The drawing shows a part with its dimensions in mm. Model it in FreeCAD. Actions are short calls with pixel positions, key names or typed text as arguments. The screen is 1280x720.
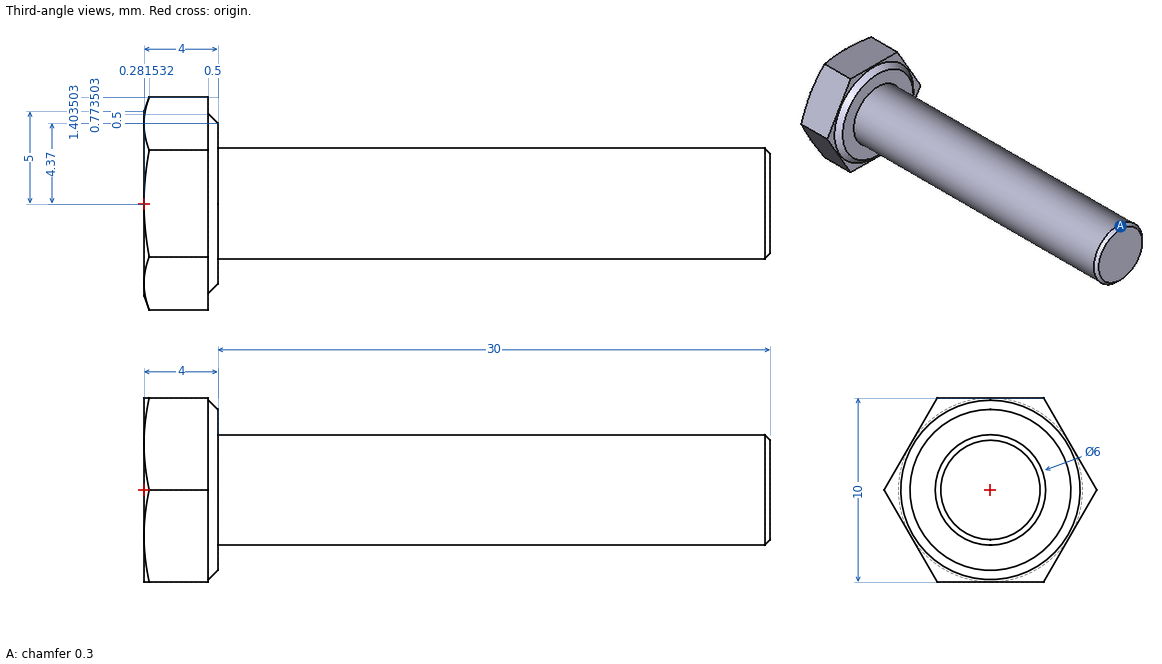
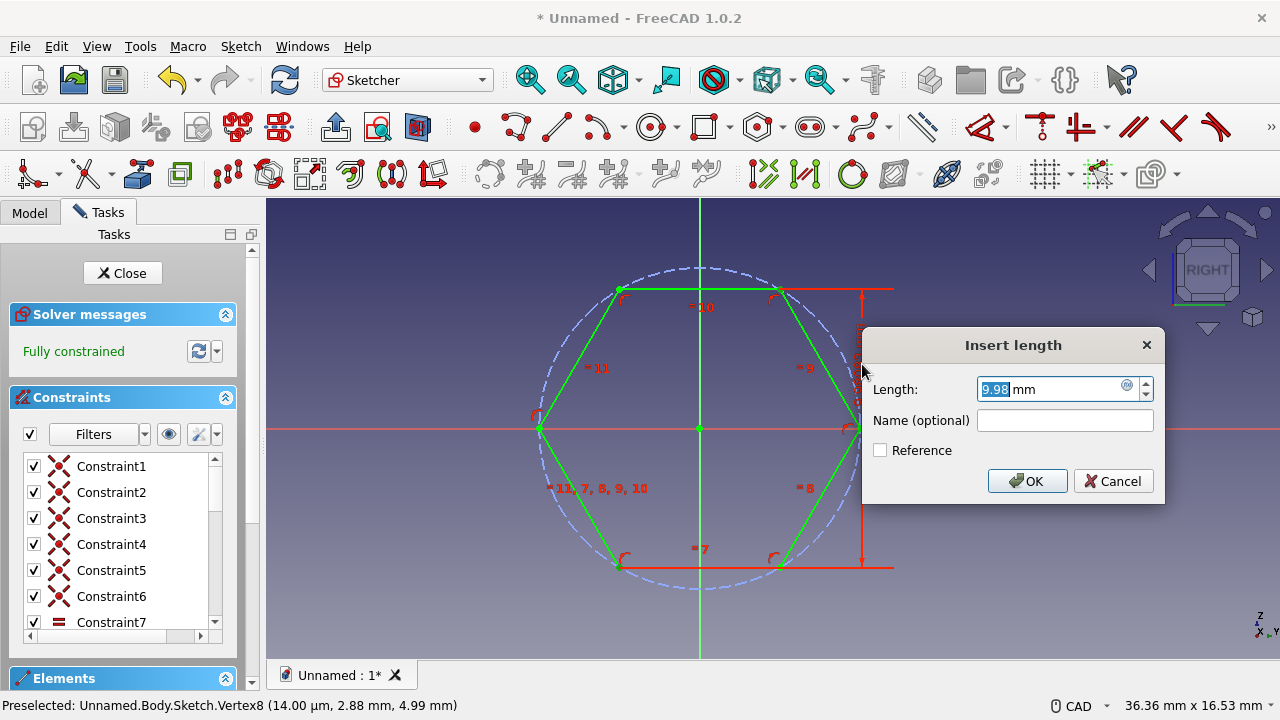
text(10)
key(Return)
key(Escape)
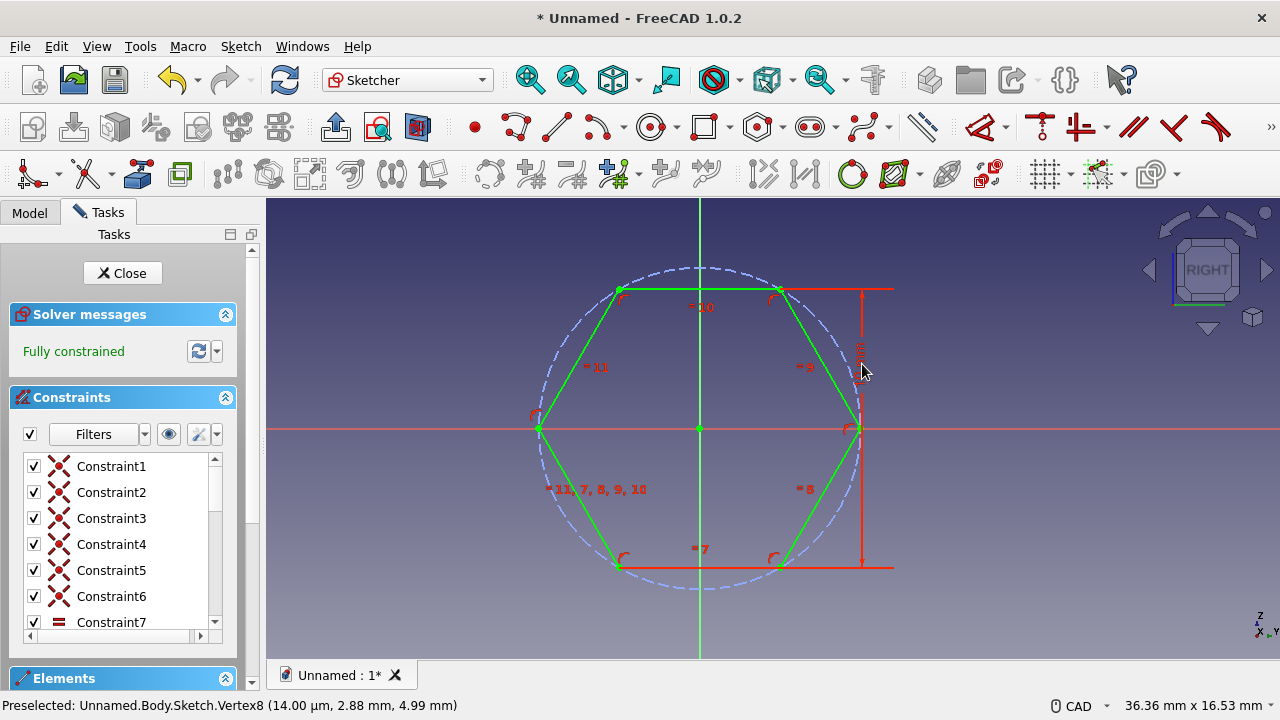
click(123, 273)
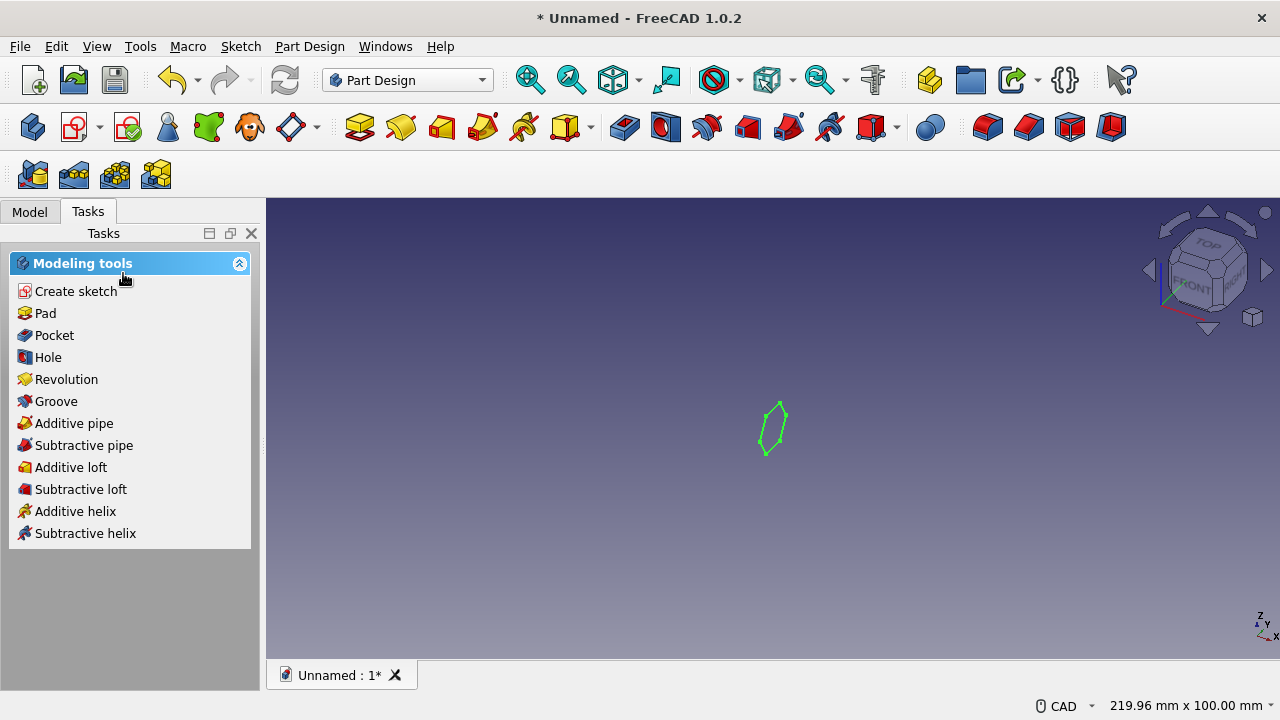
click(360, 128)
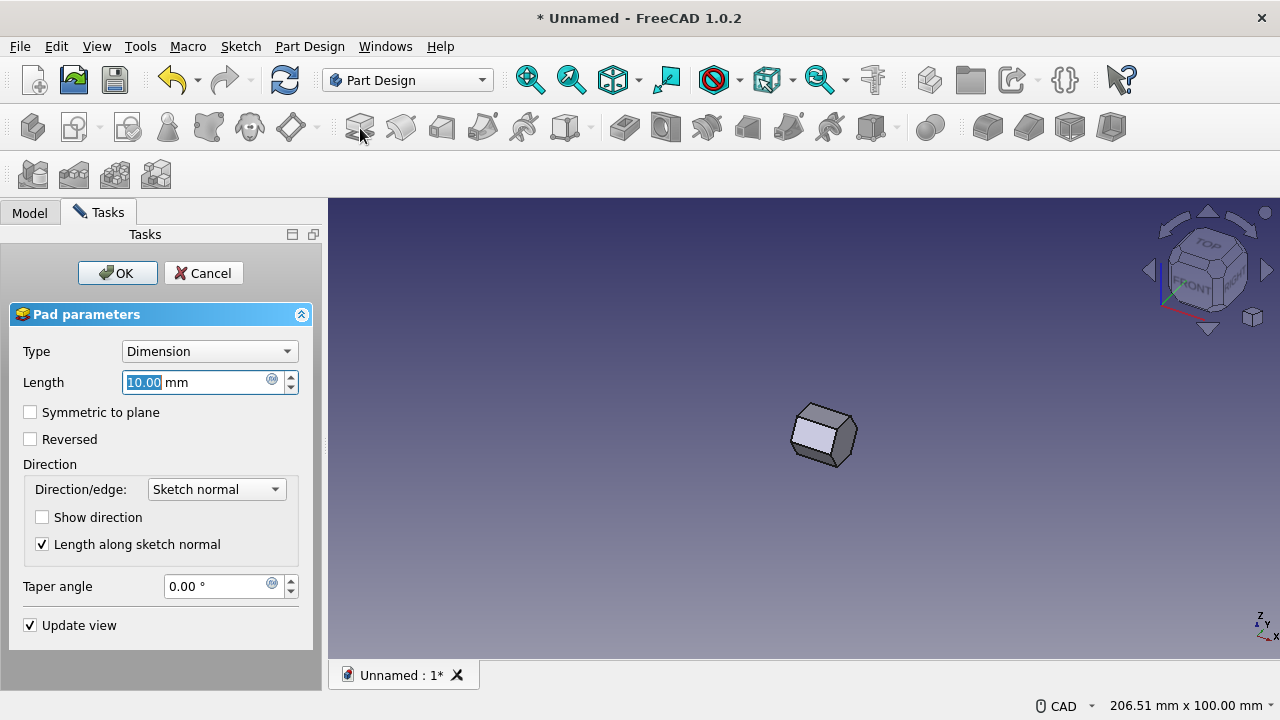
text(4)
key(Tab)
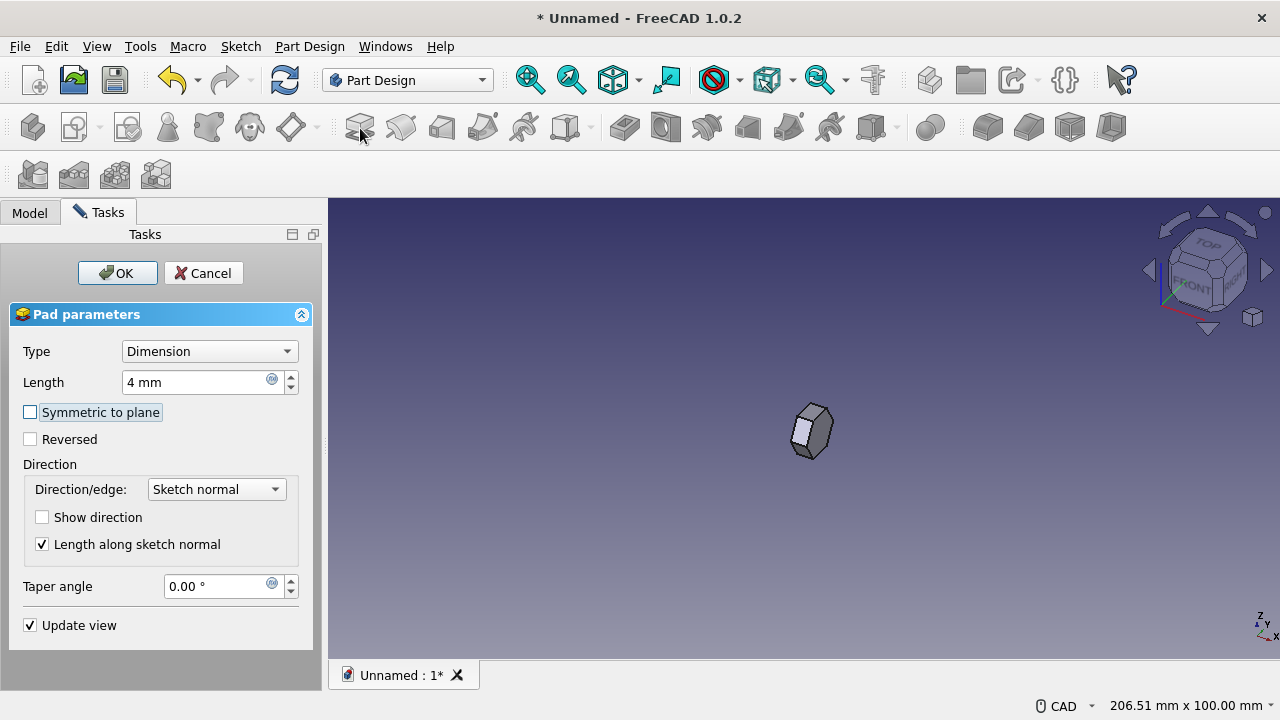
click(118, 273)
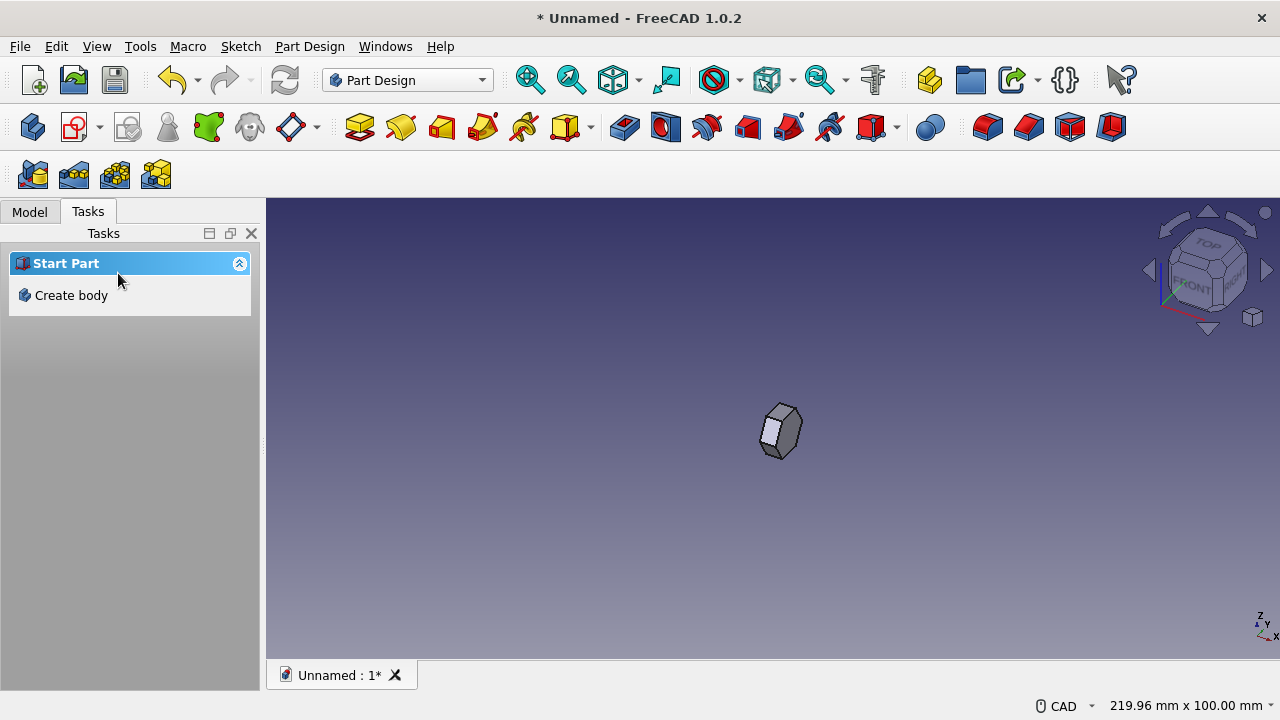
click(531, 80)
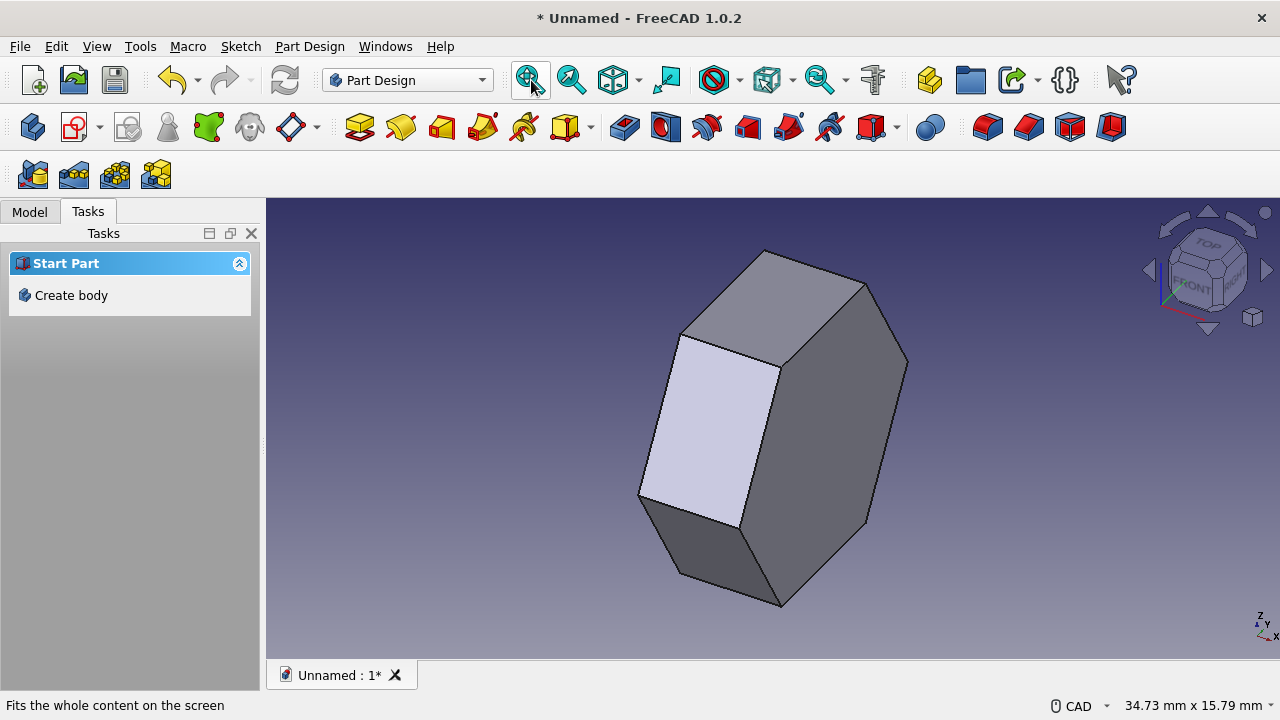
click(74, 128)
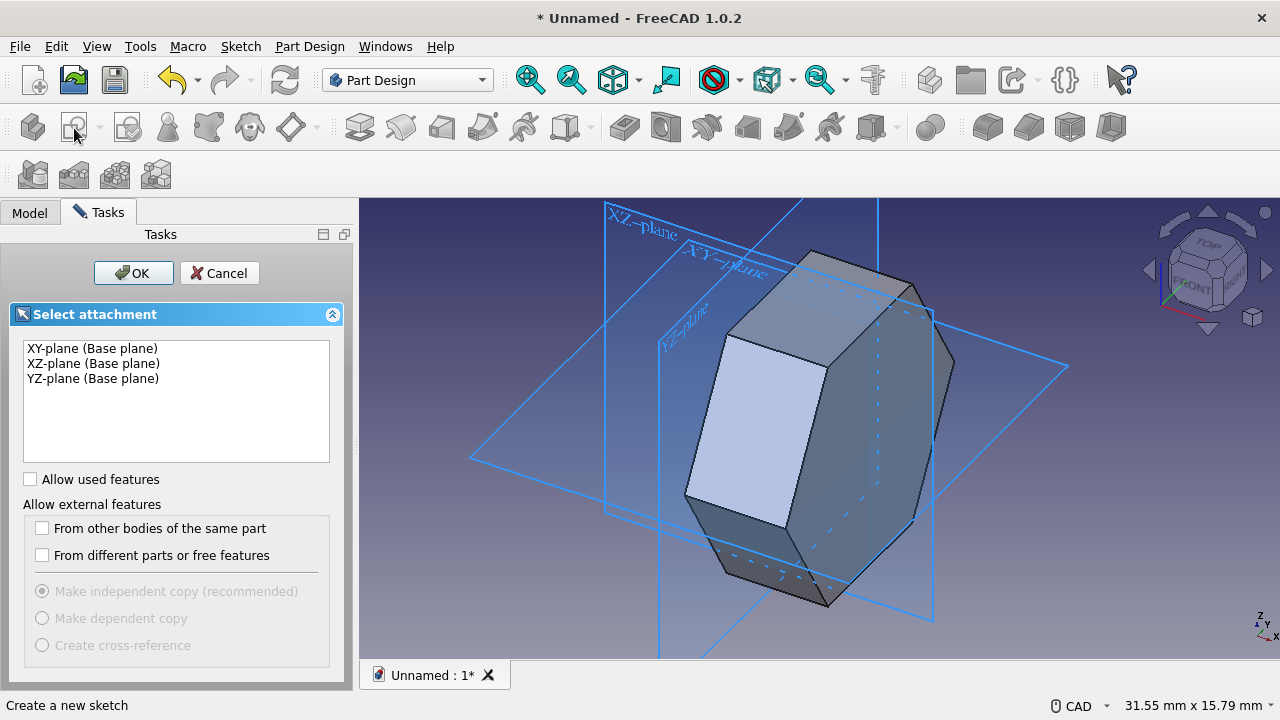
click(84, 348)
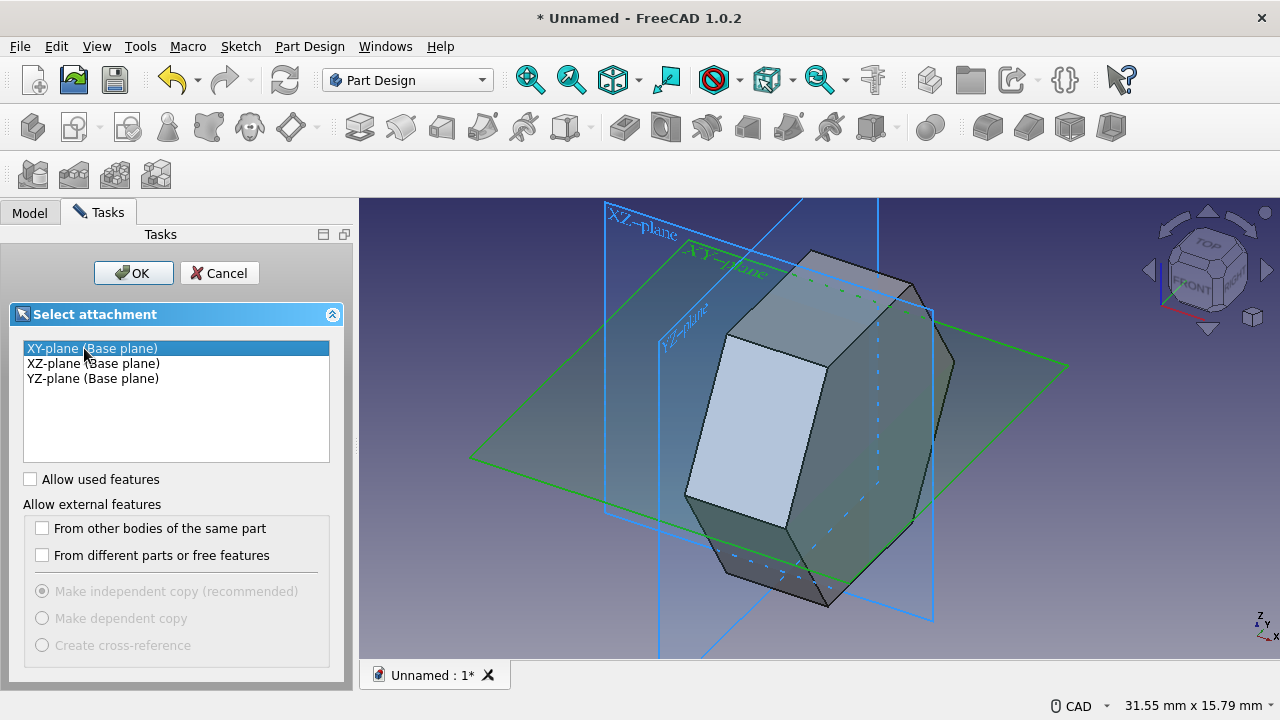
click(134, 273)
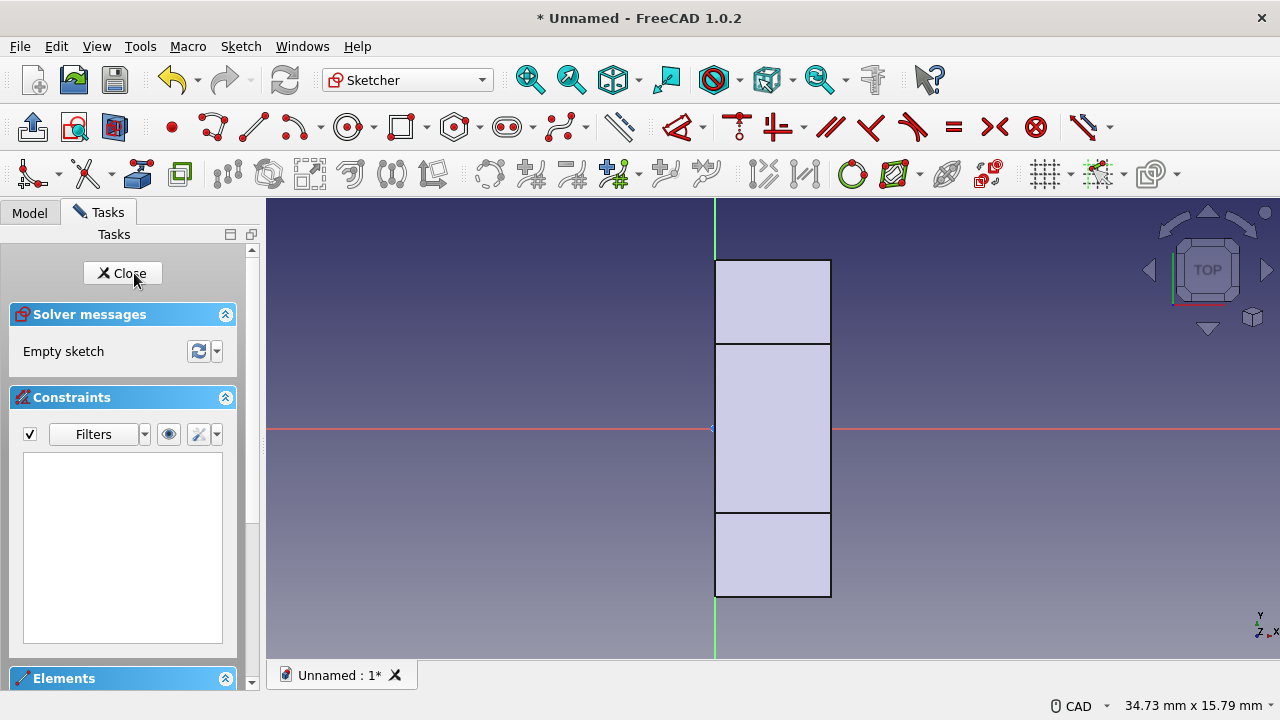
click(115, 128)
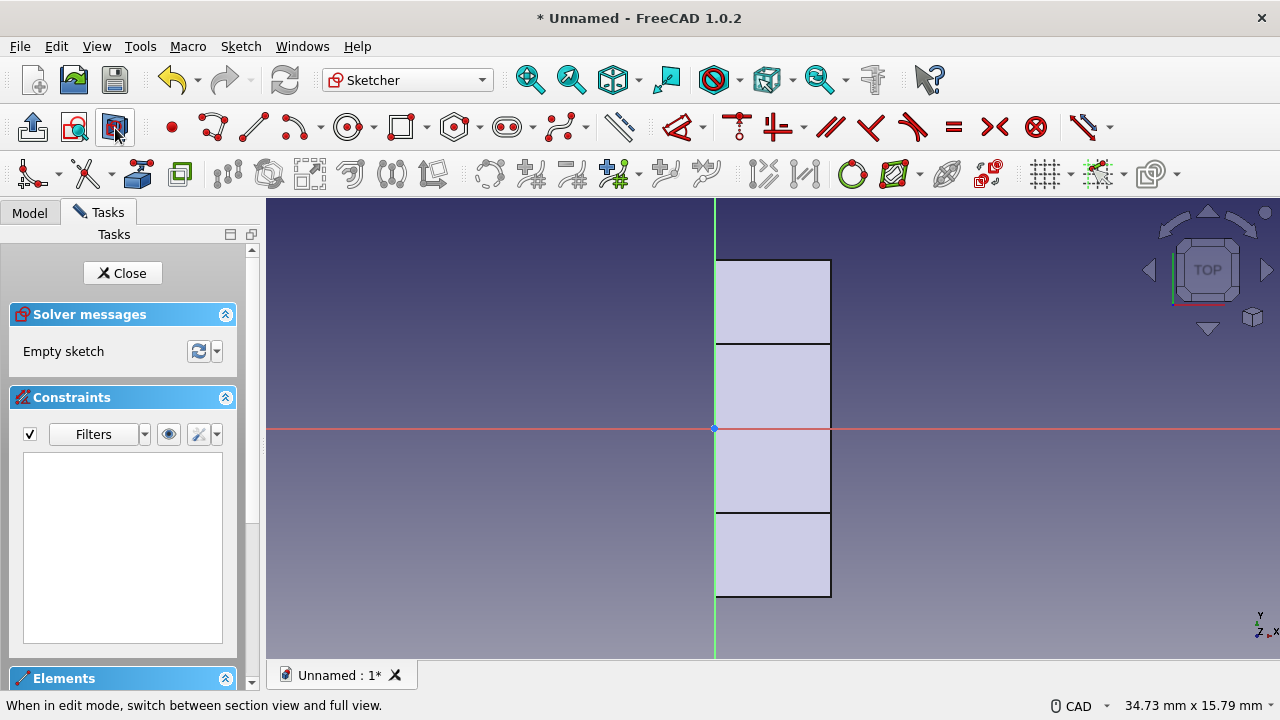
scroll(843, 257, up, 10)